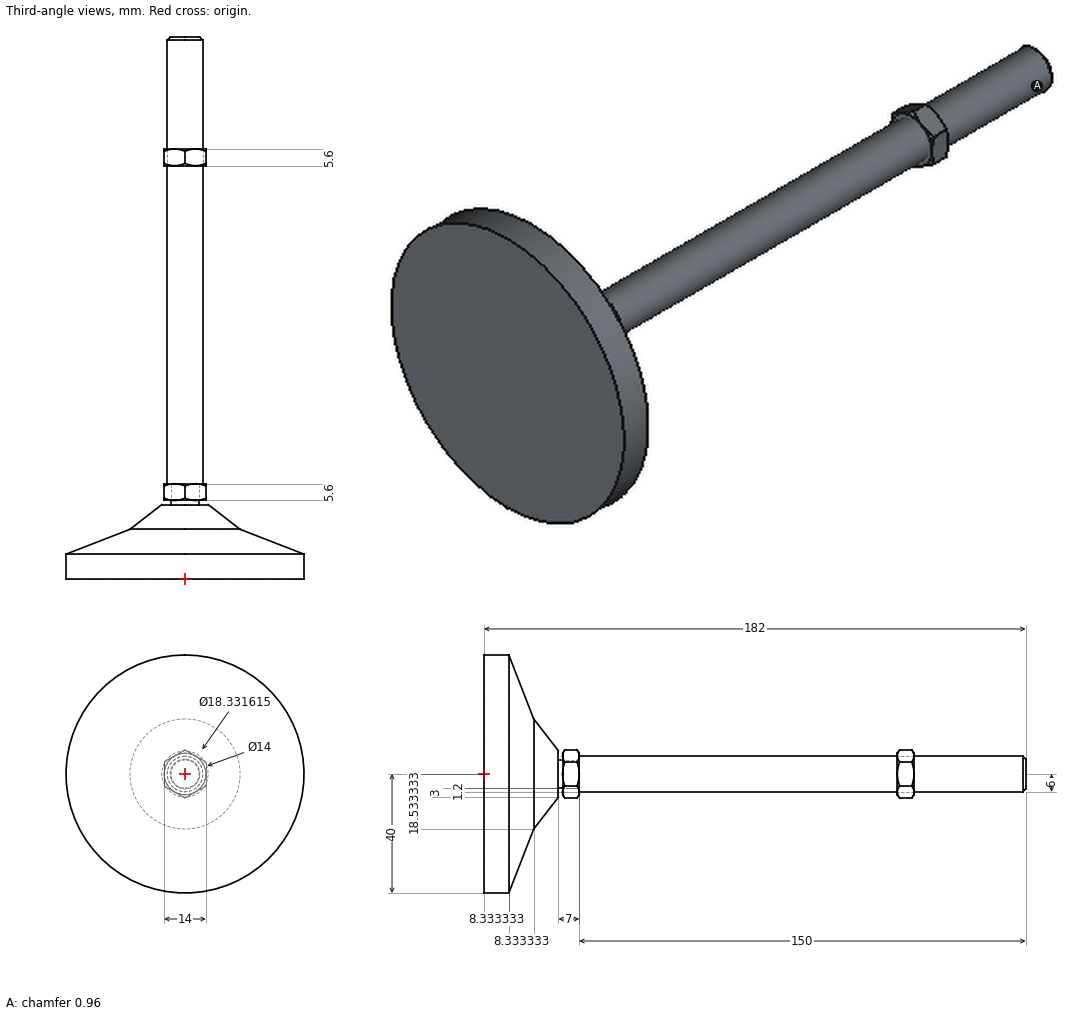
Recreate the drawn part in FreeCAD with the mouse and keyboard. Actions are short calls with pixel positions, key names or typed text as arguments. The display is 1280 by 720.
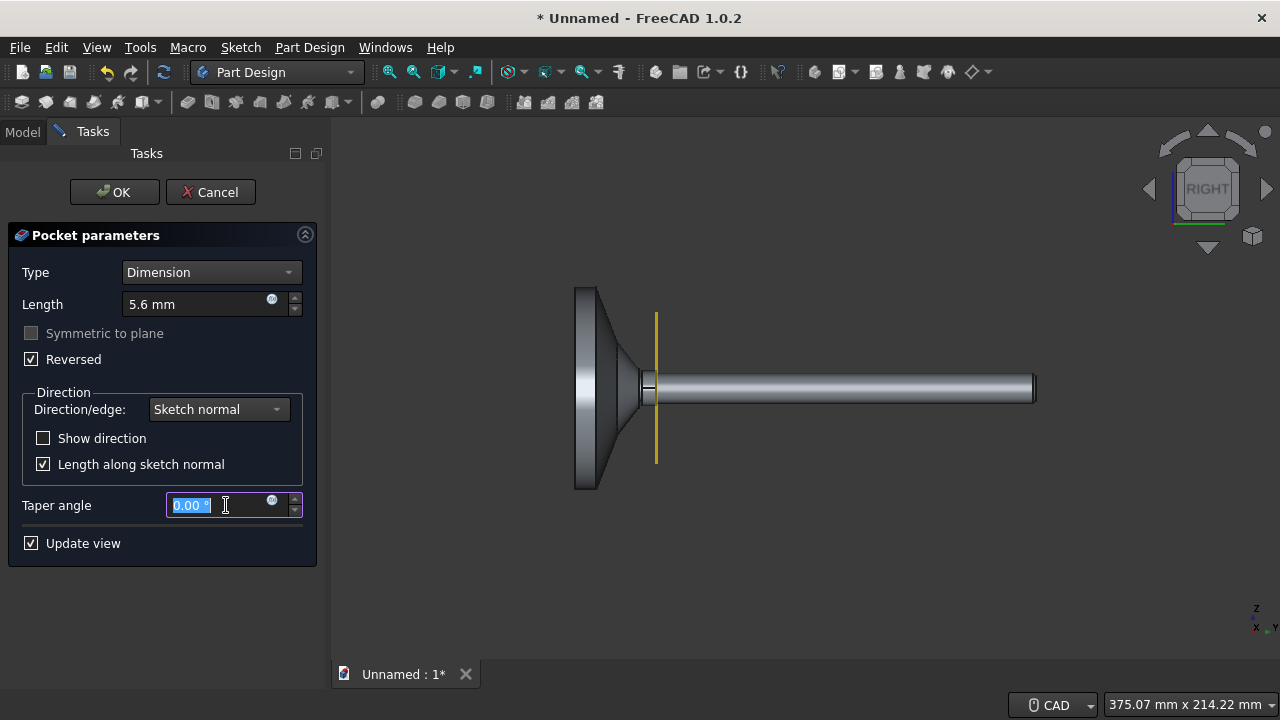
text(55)
key(Tab)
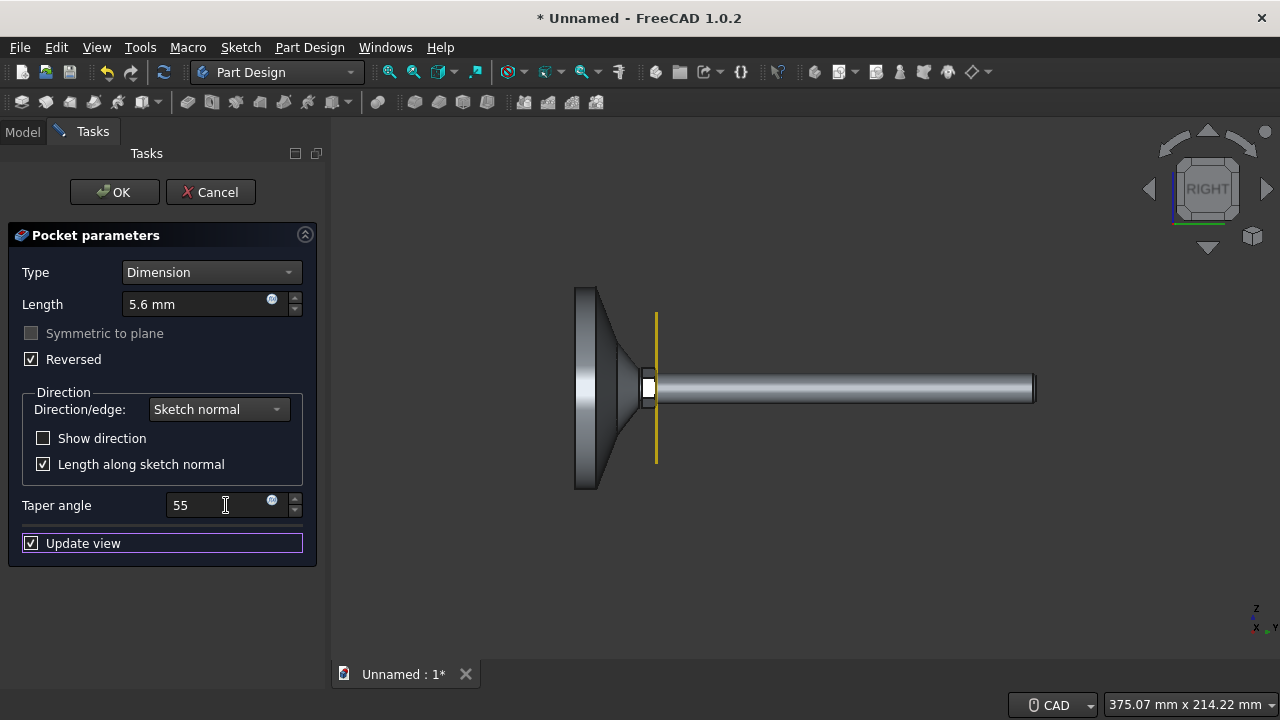
click(115, 192)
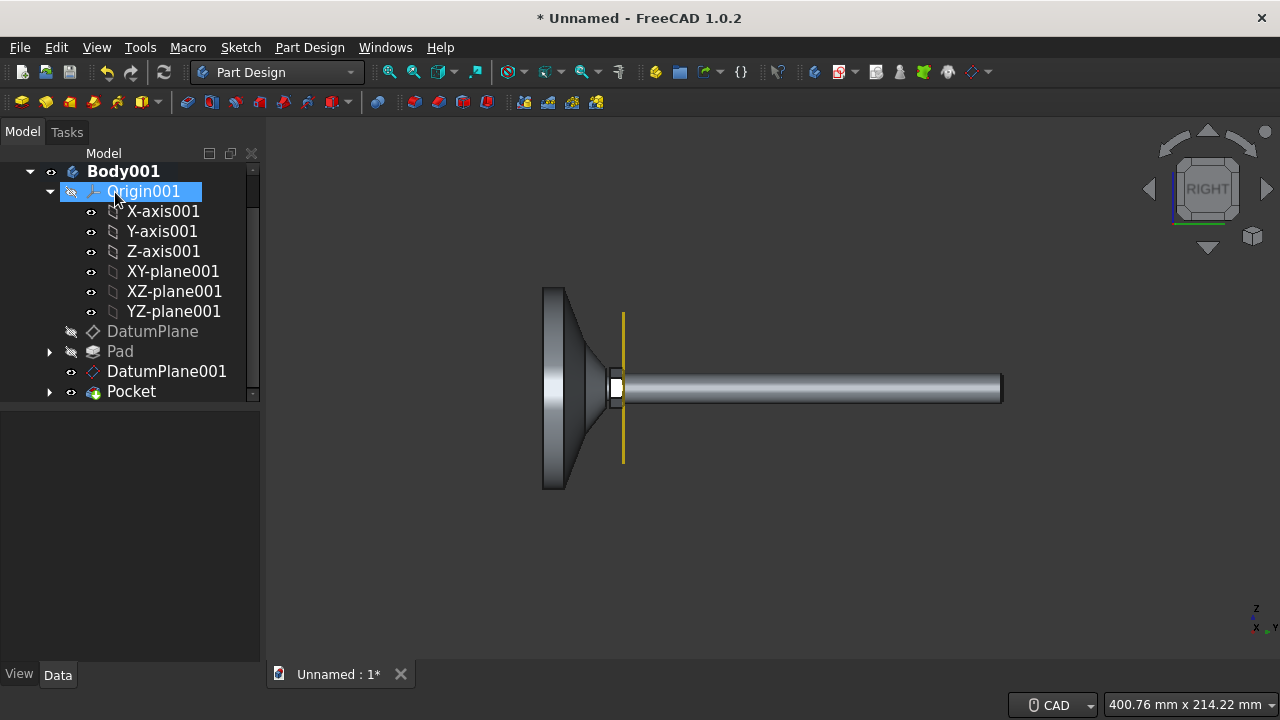
click(116, 372)
key(space)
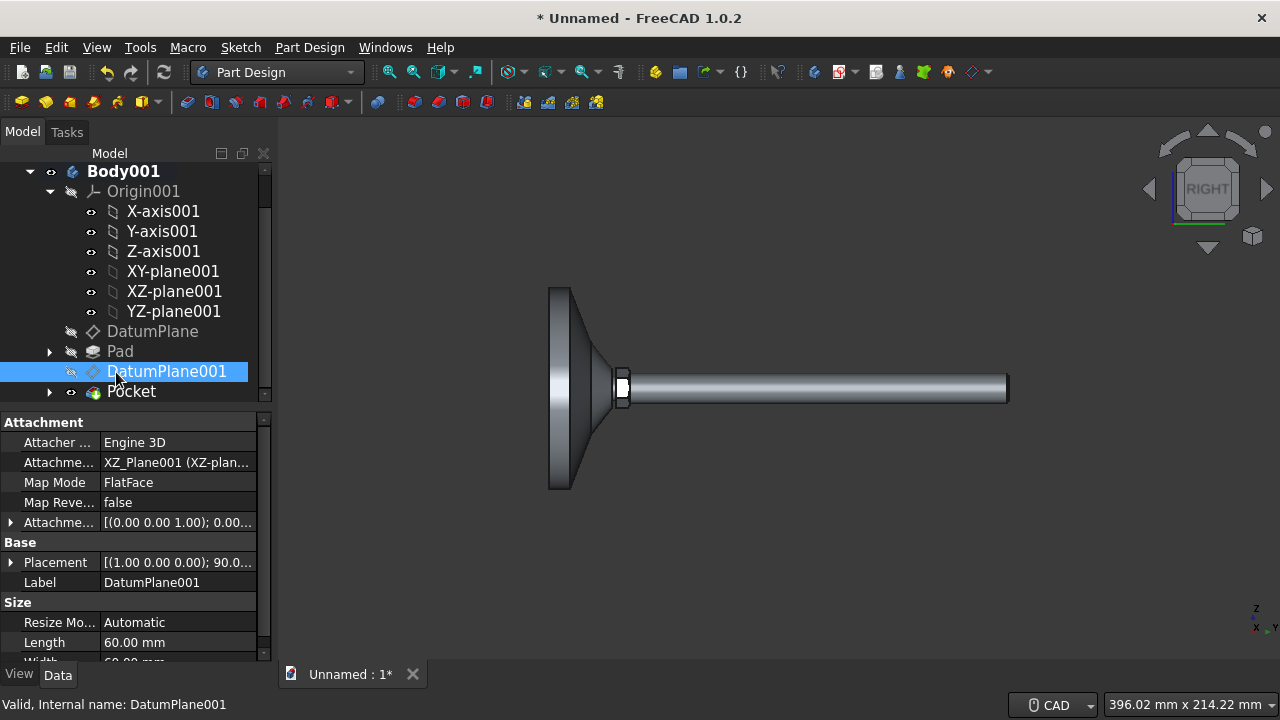
click(390, 72)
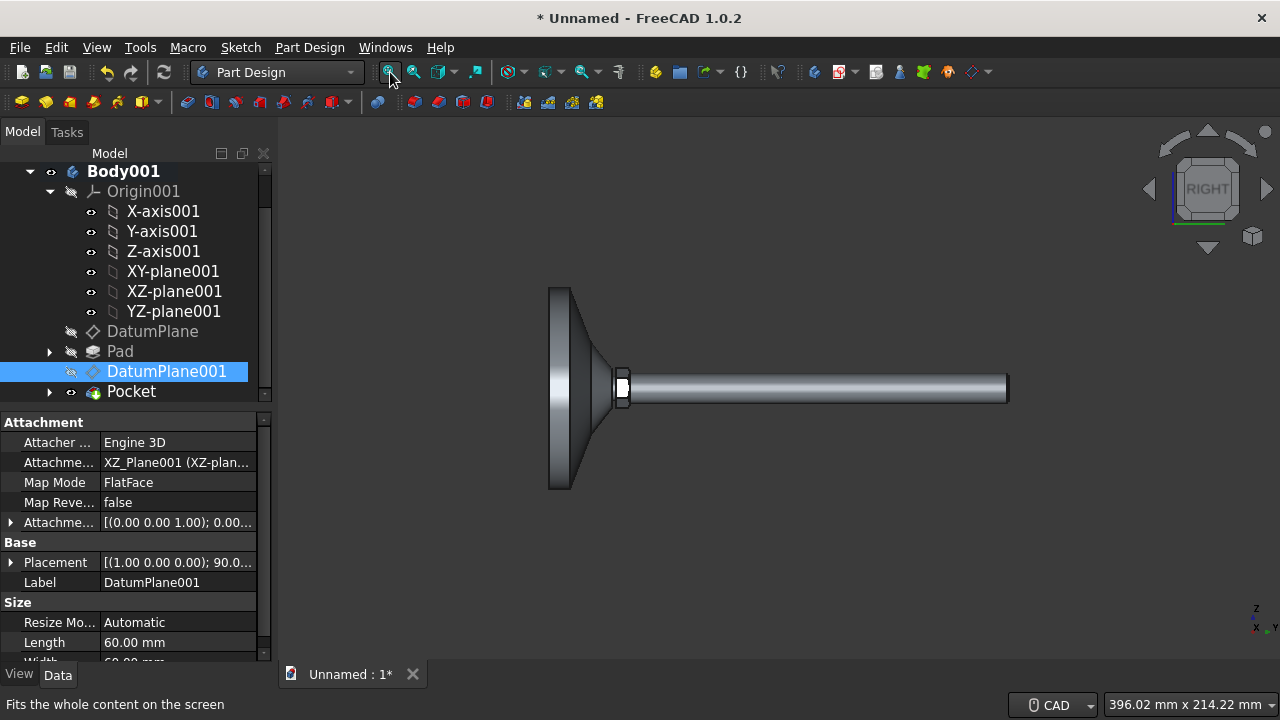
key(0)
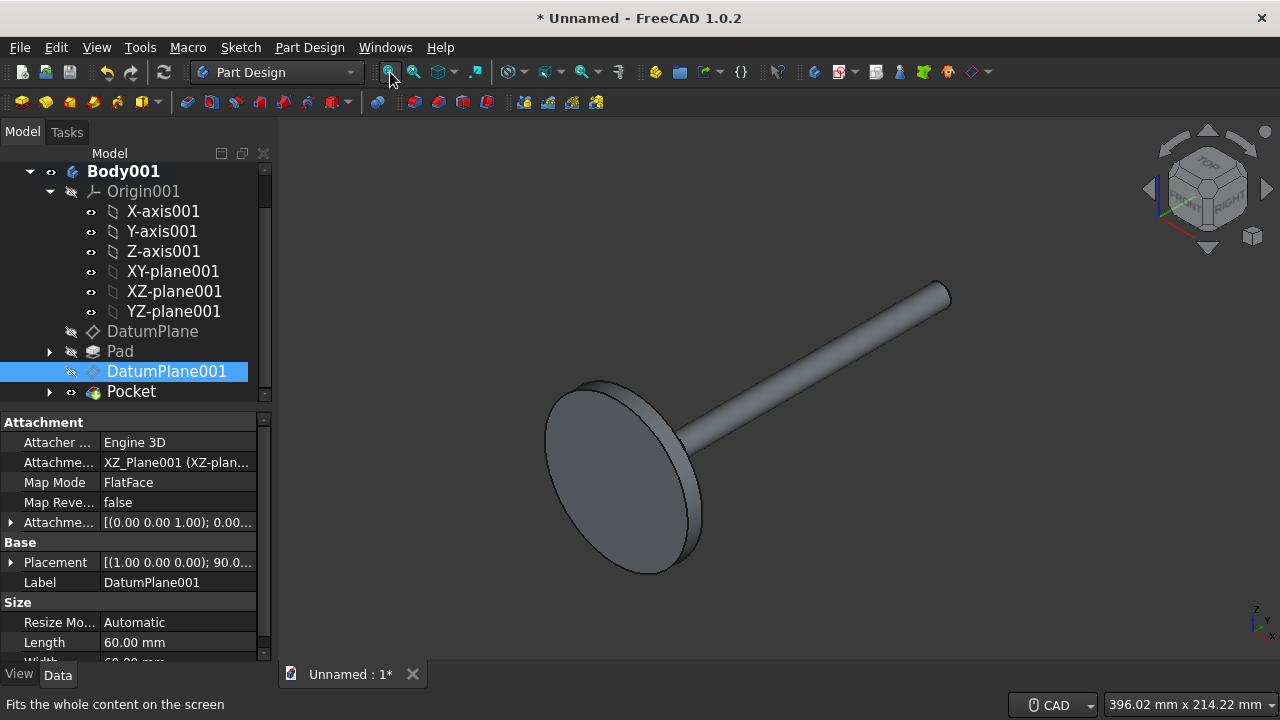
click(390, 72)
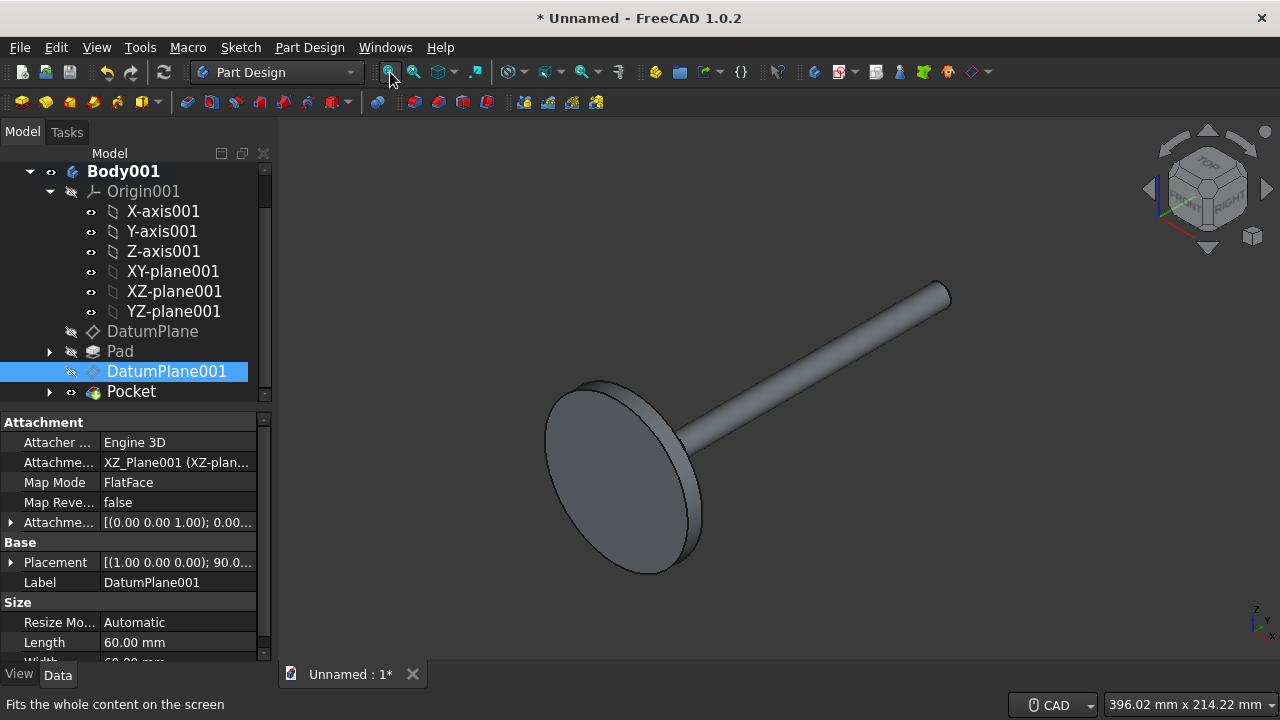
key(1)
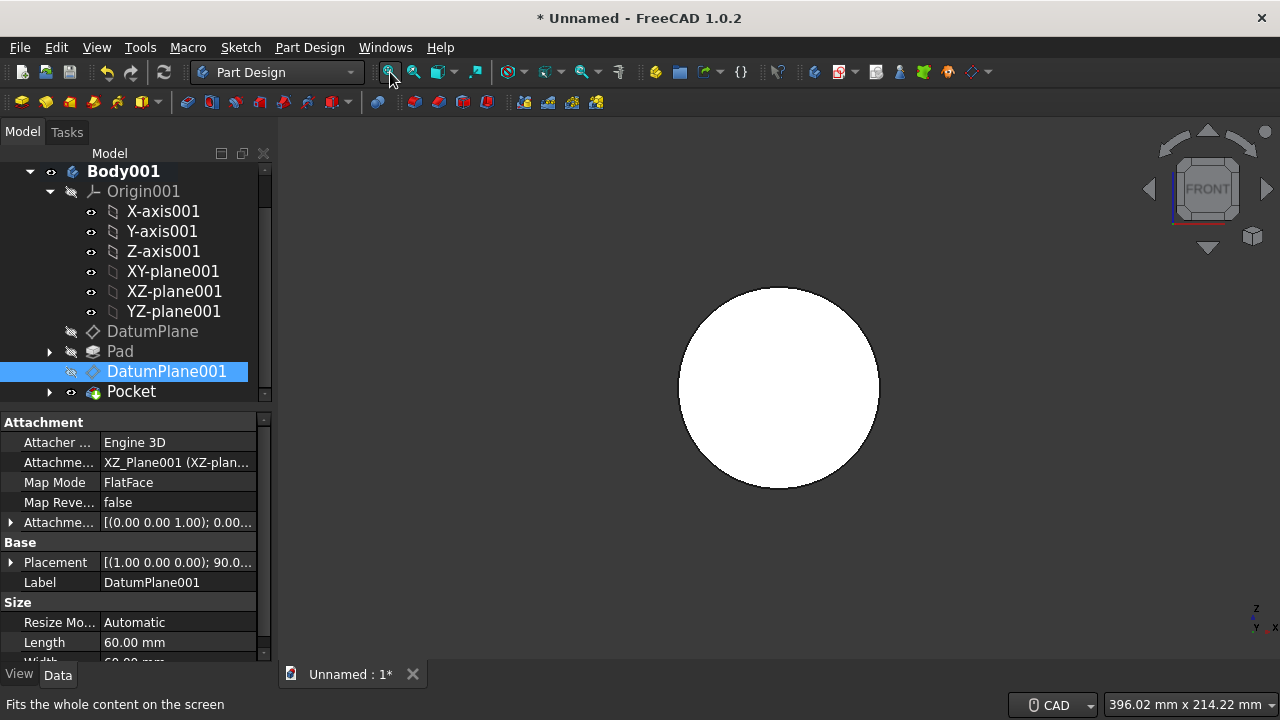
key(v)
key(f)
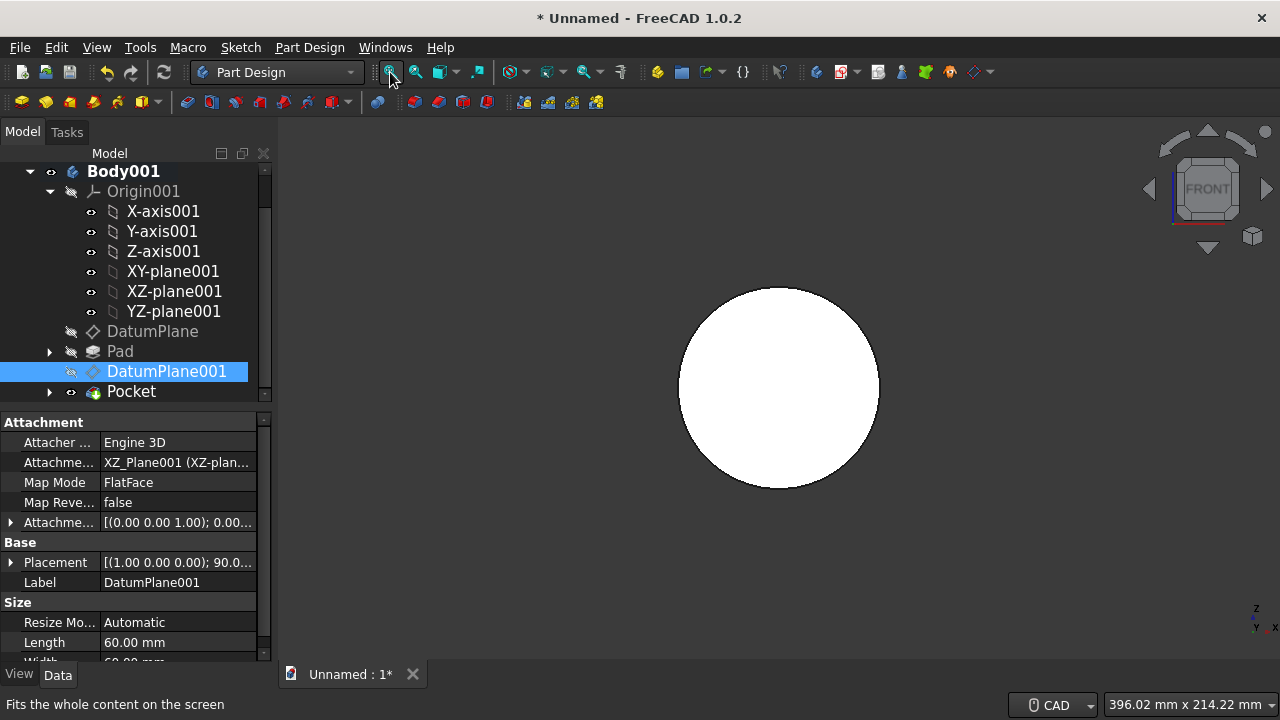
key(2)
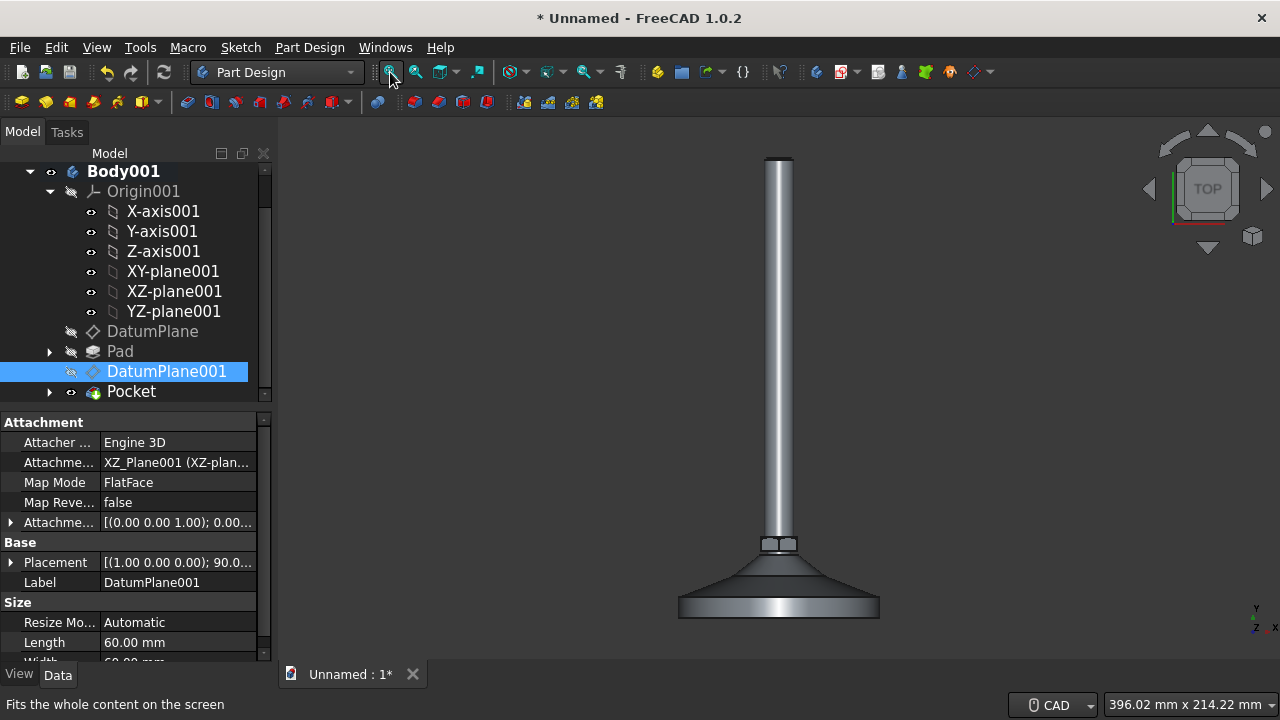
click(392, 72)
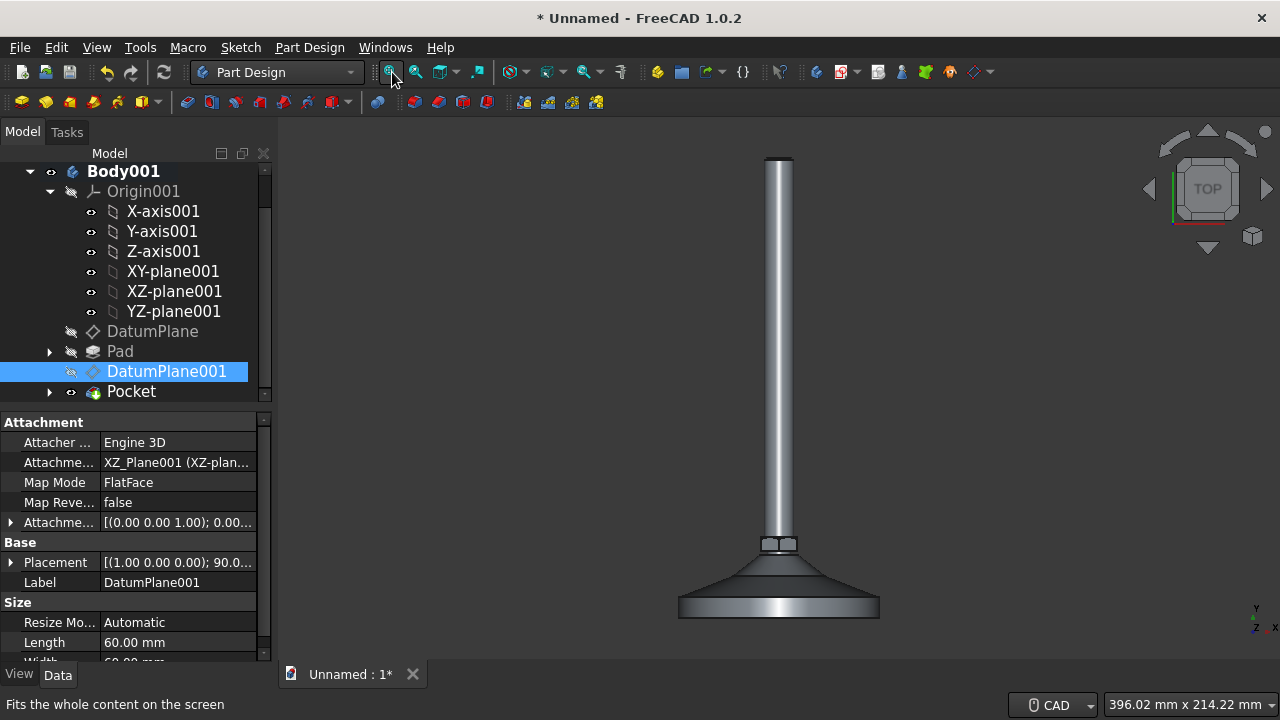
click(136, 292)